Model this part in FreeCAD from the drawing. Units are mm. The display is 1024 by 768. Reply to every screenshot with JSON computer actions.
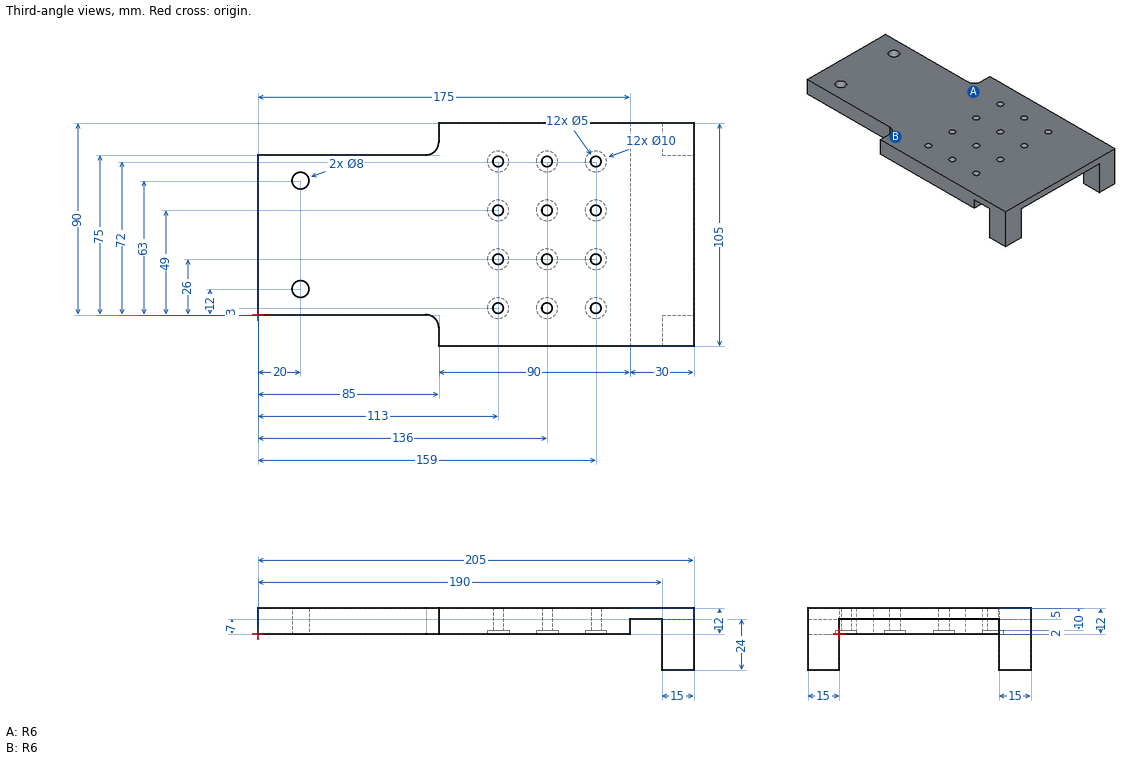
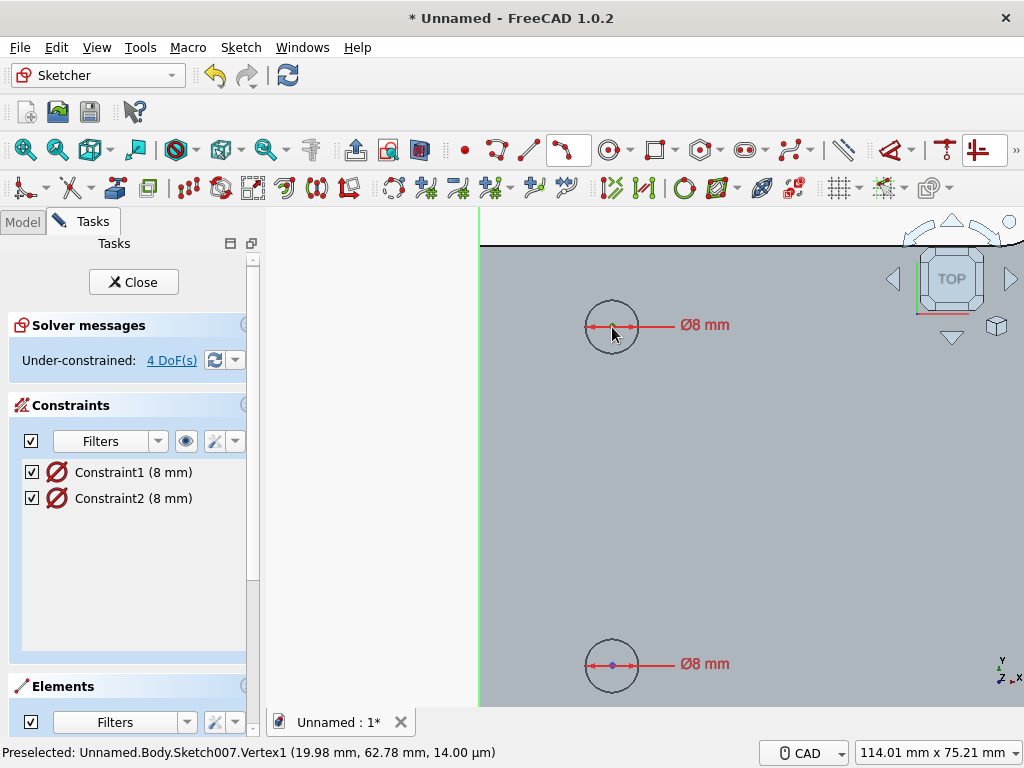
{"action": "left_click", "coordinate": [612, 666]}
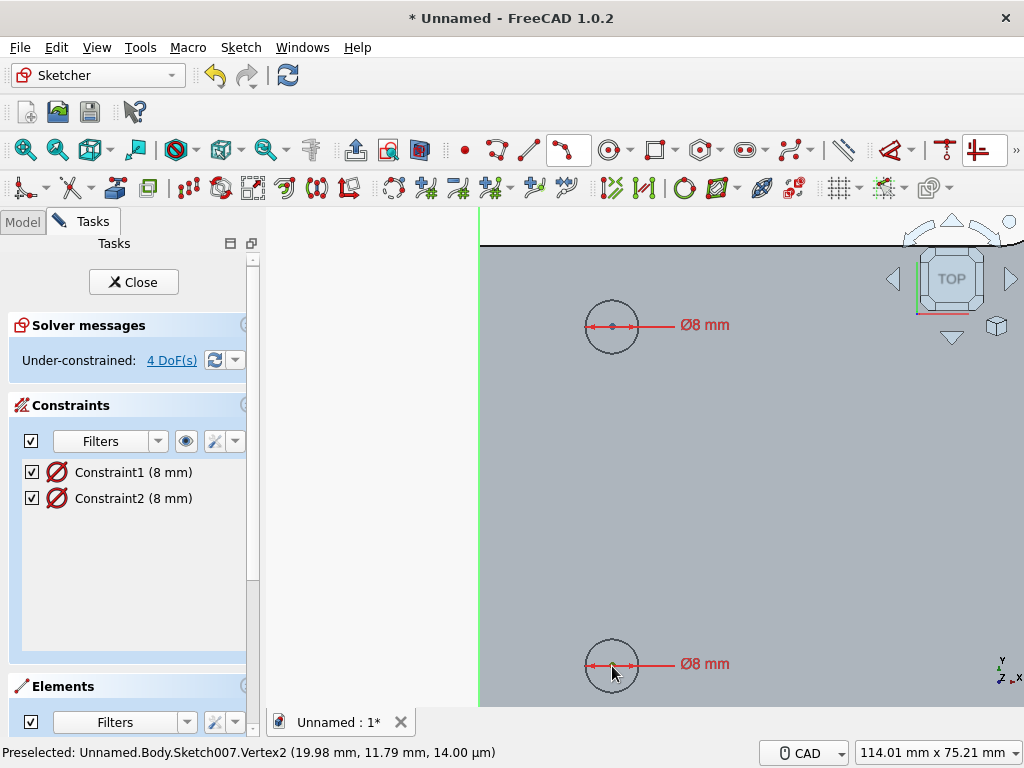
{"action": "left_click", "coordinate": [1002, 150]}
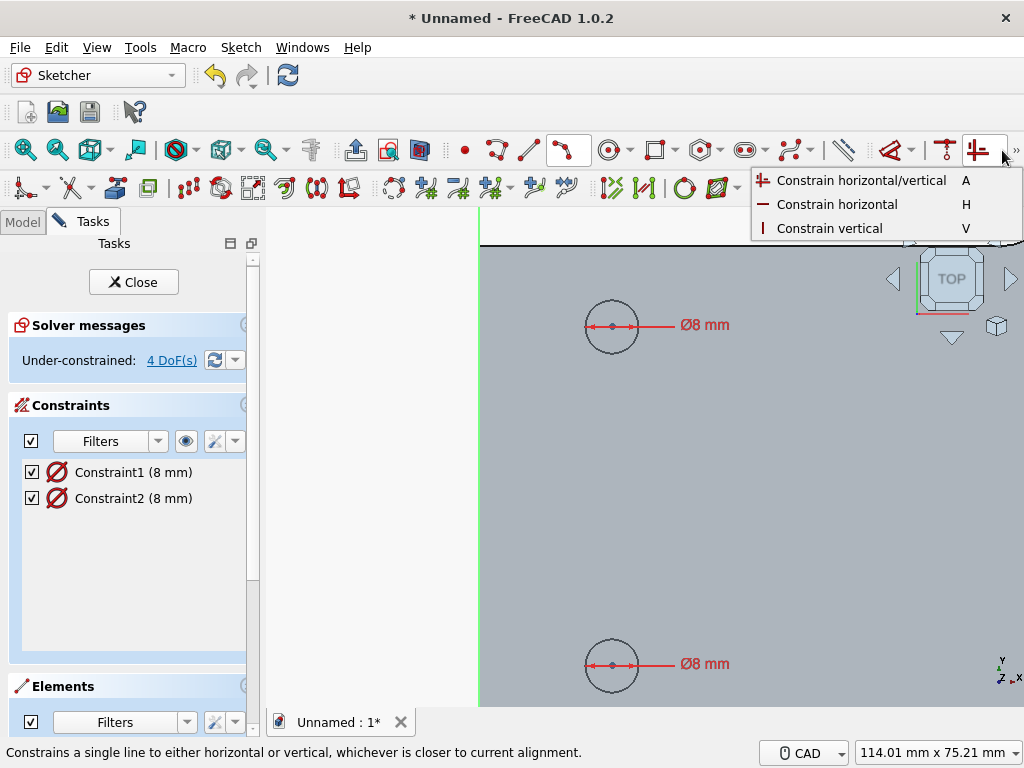
{"action": "left_click", "coordinate": [887, 228]}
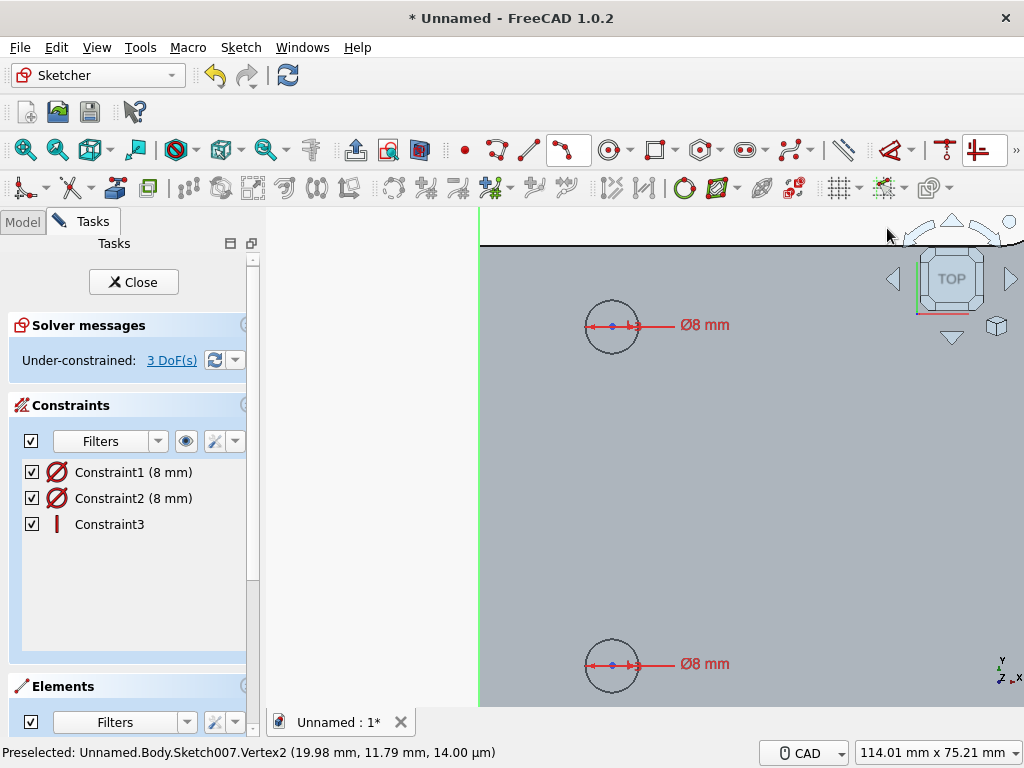
{"action": "left_click", "coordinate": [890, 150]}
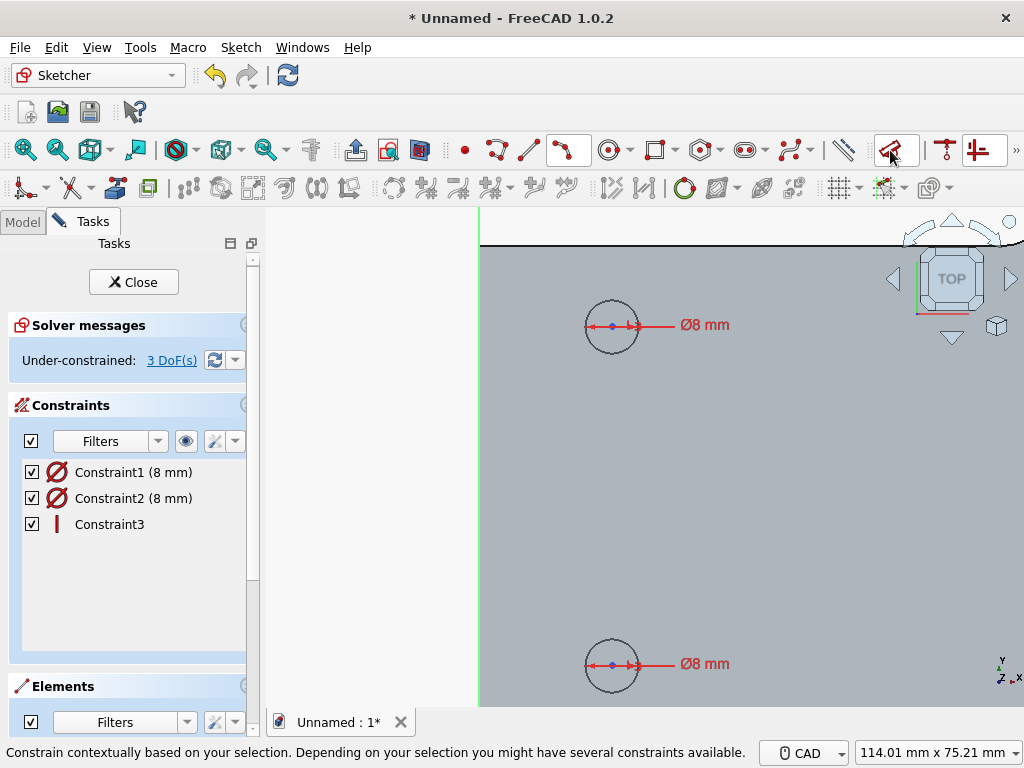
{"action": "left_click", "coordinate": [612, 327]}
{"action": "left_click", "coordinate": [546, 293]}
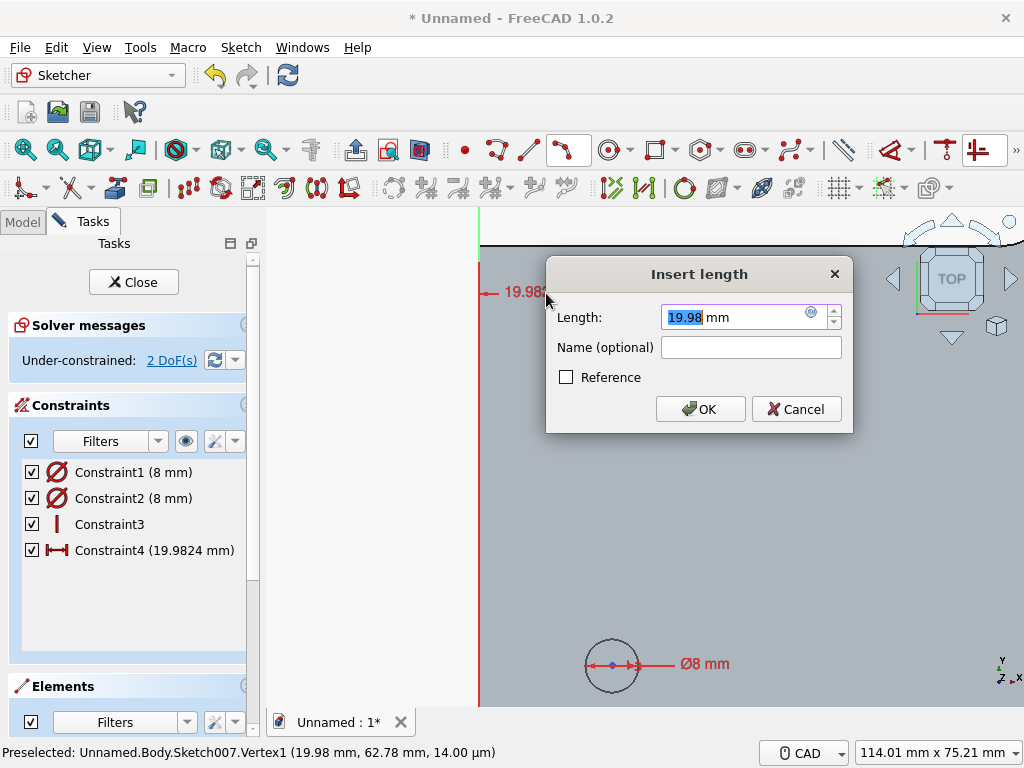
{"action": "type", "text": "20"}
{"action": "key", "text": "Return"}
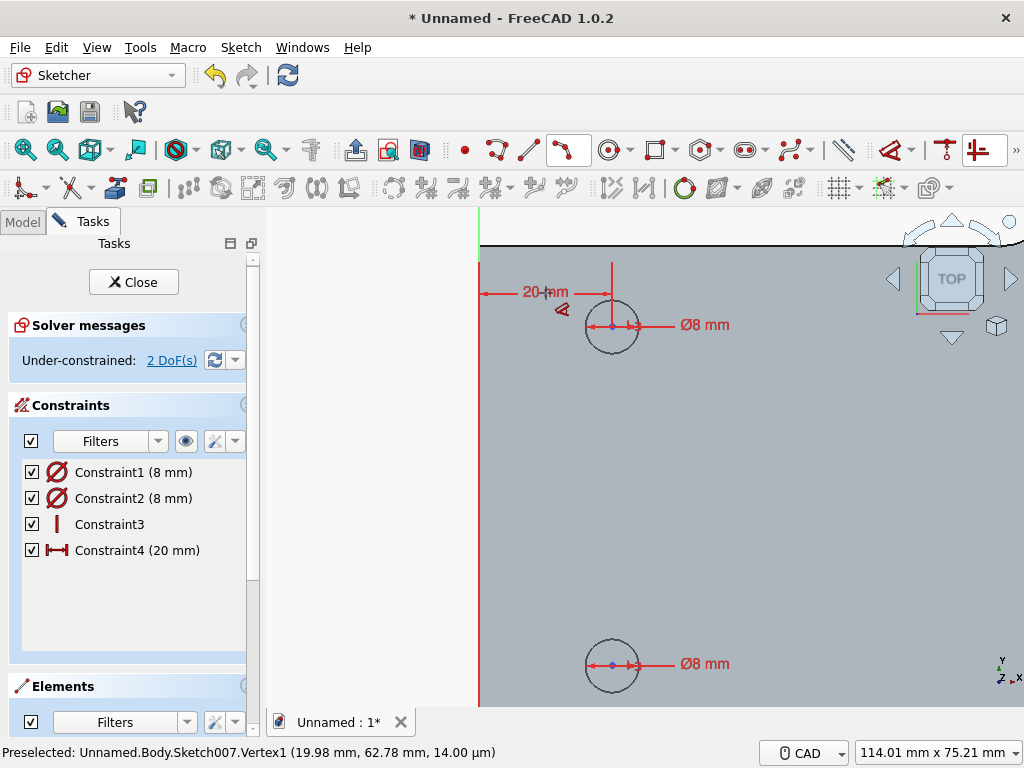
{"action": "left_click", "coordinate": [612, 327]}
{"action": "left_click", "coordinate": [445, 503]}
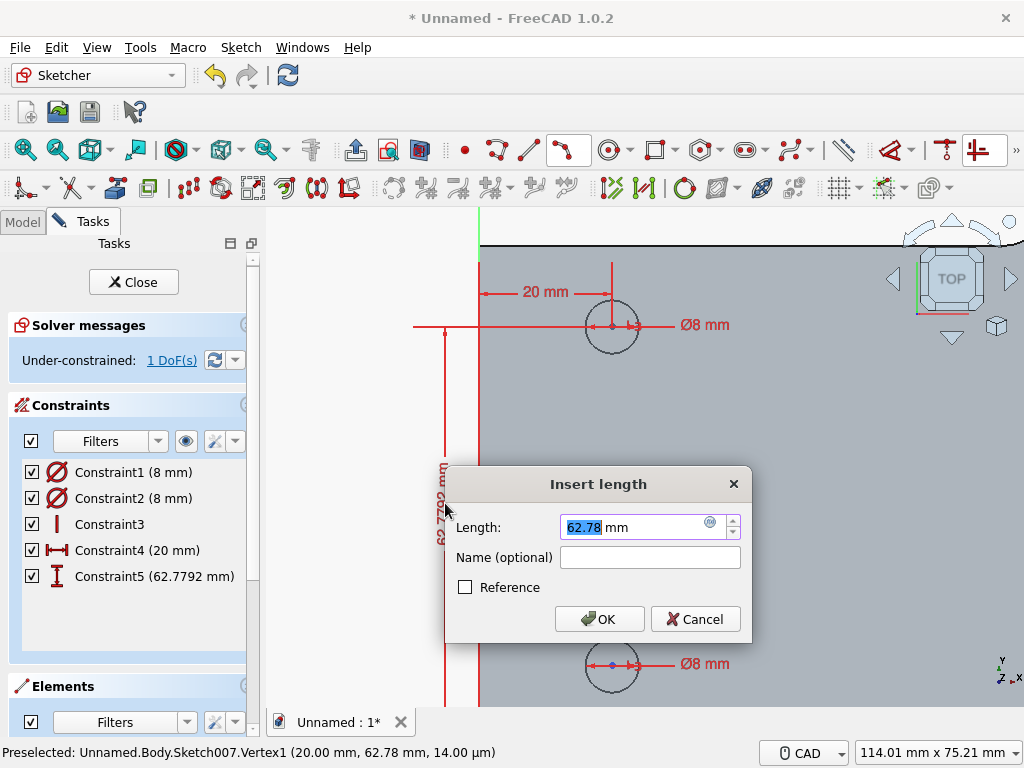
{"action": "type", "text": "63"}
{"action": "key", "text": "Return"}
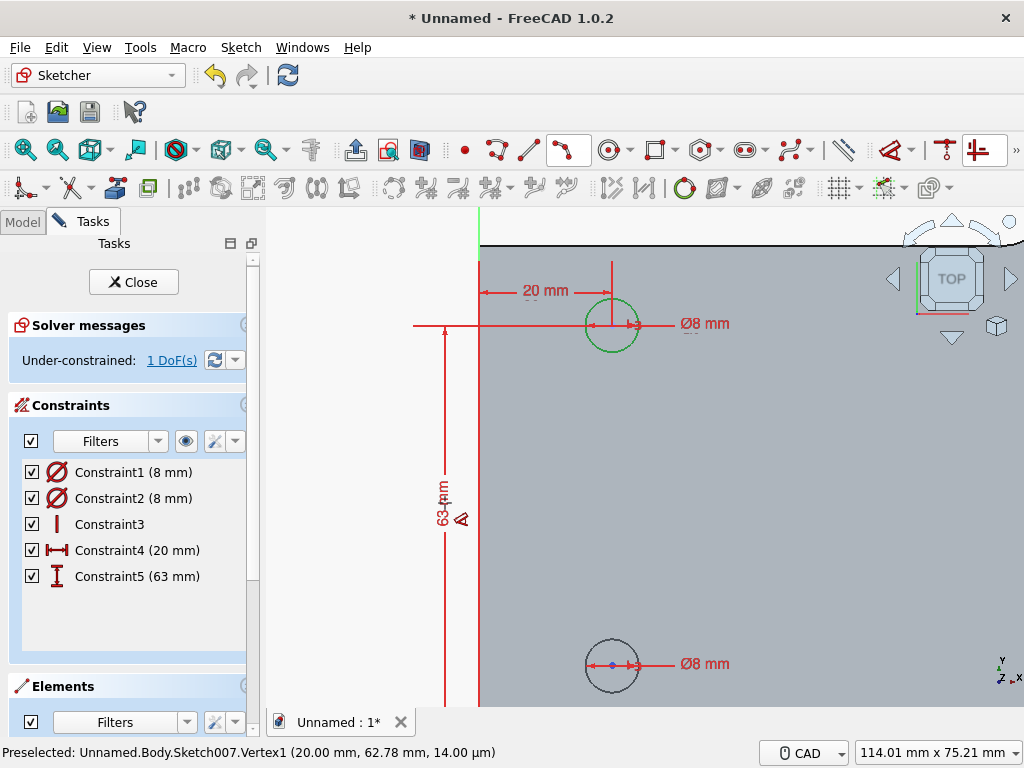
{"action": "left_click", "coordinate": [612, 666]}
{"action": "left_click", "coordinate": [445, 673]}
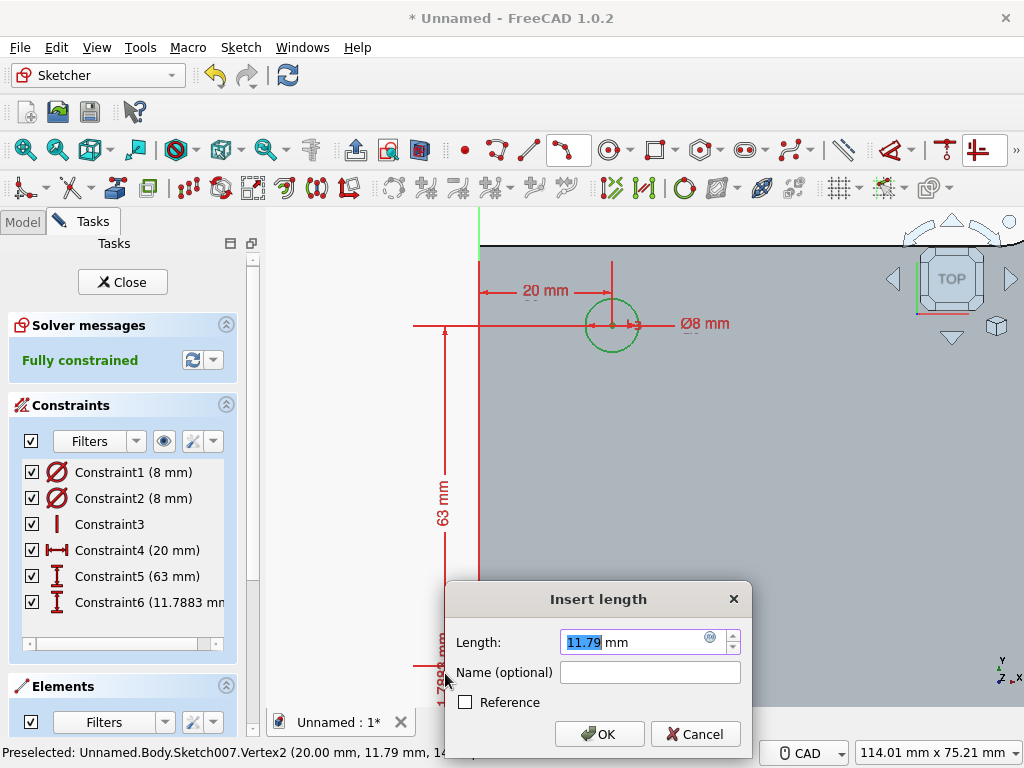
{"action": "type", "text": "12"}
{"action": "key", "text": "Return"}
{"action": "key", "text": "Escape"}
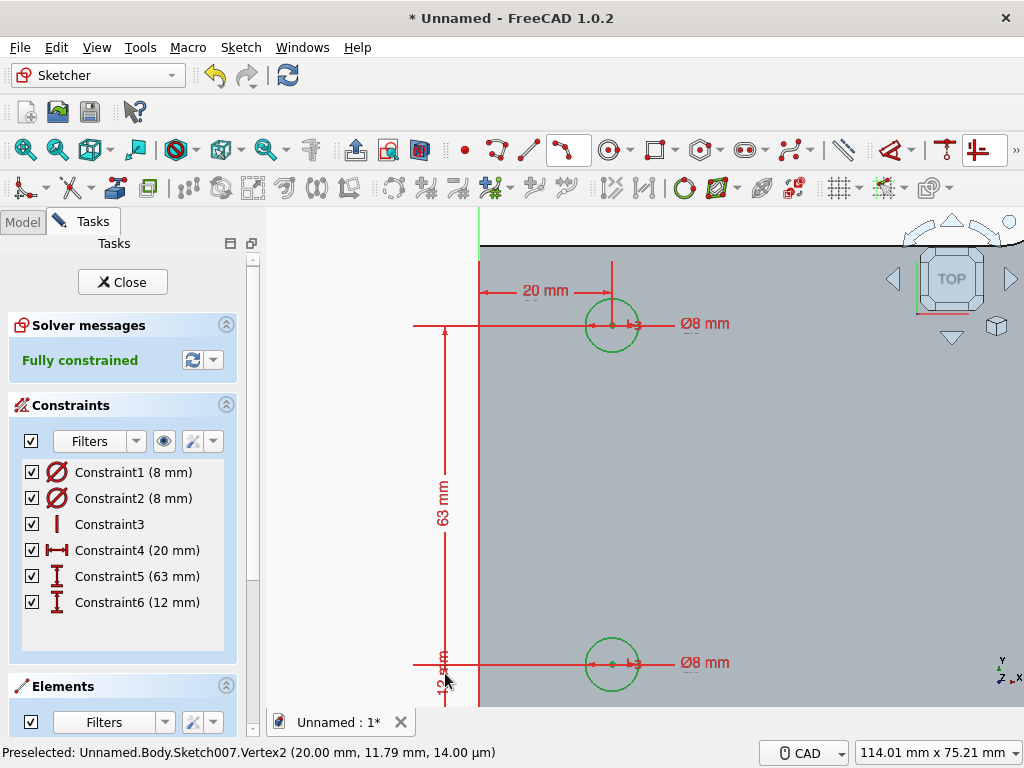
{"action": "left_click", "coordinate": [123, 282]}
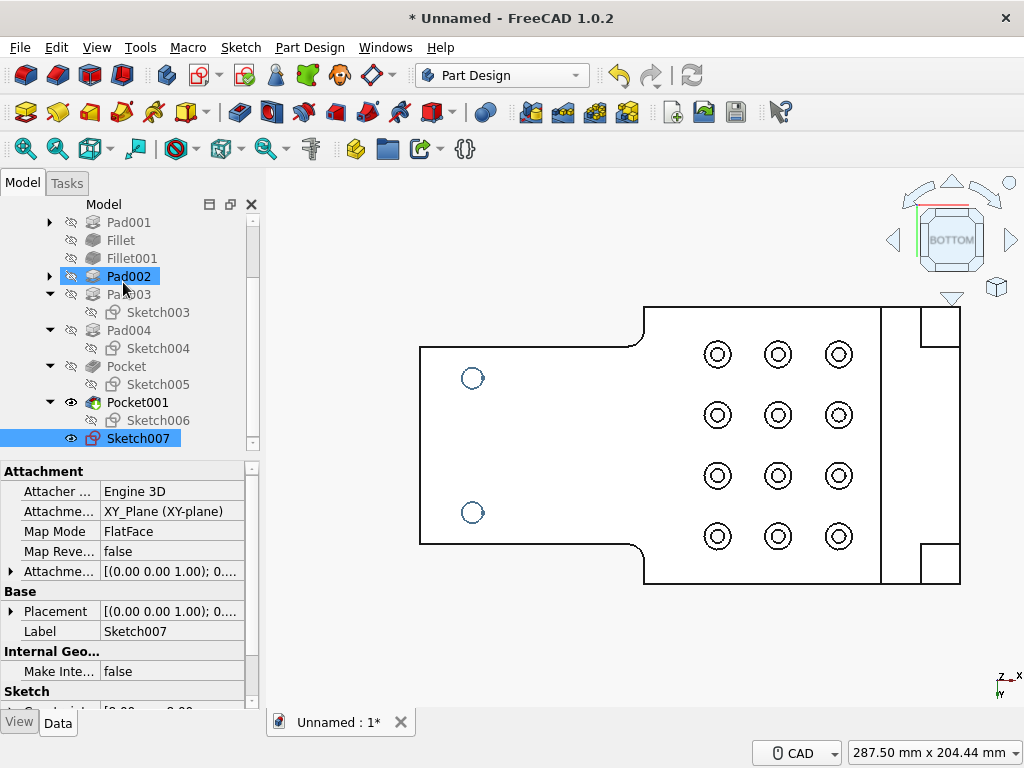
{"action": "left_click", "coordinate": [240, 112]}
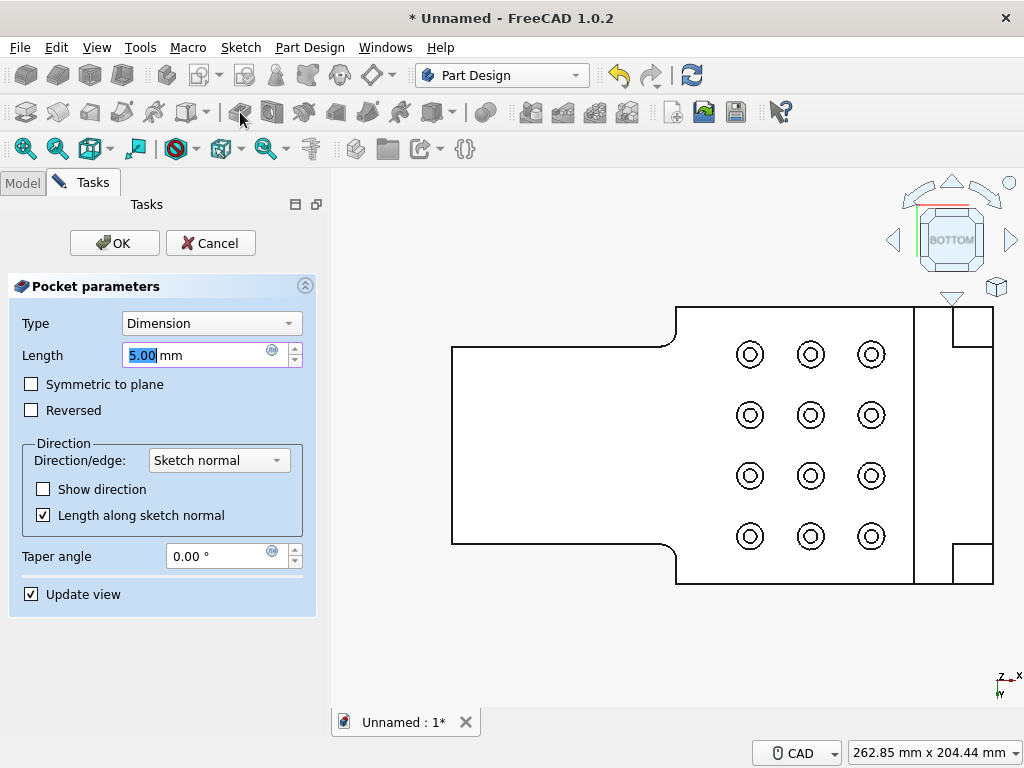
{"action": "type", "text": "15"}
{"action": "key", "text": "Tab"}